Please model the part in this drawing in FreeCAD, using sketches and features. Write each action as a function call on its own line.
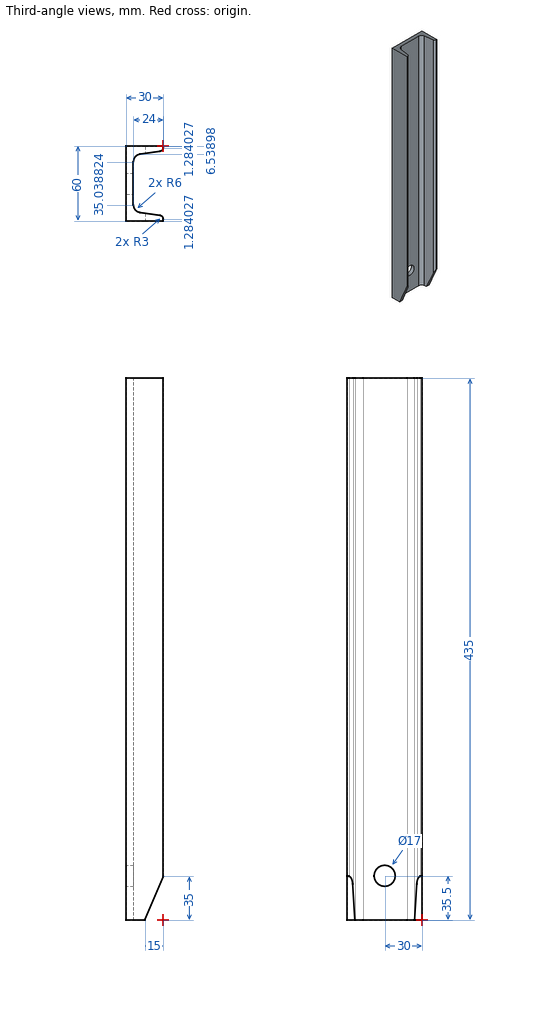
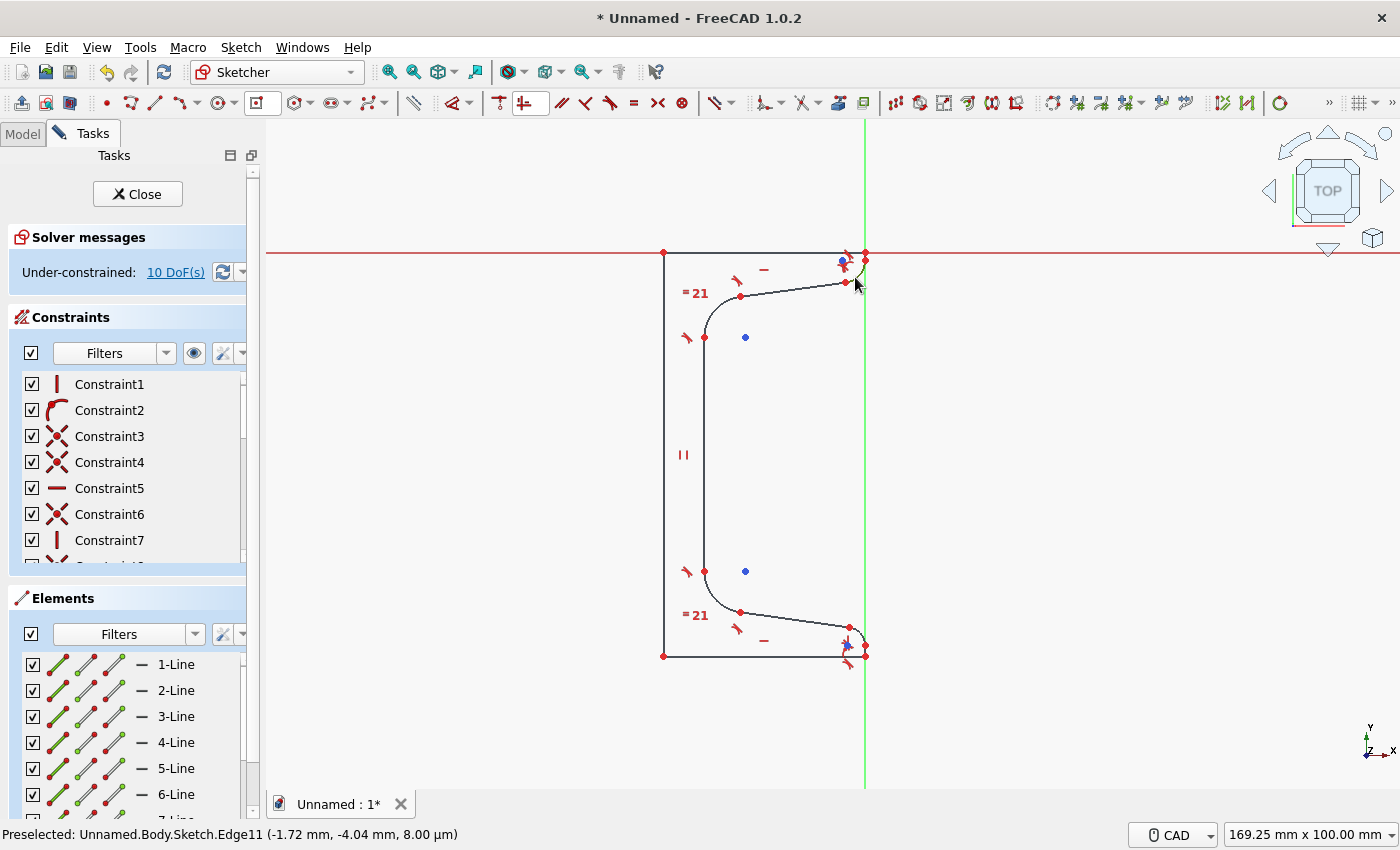
scroll(863, 638, up, 3)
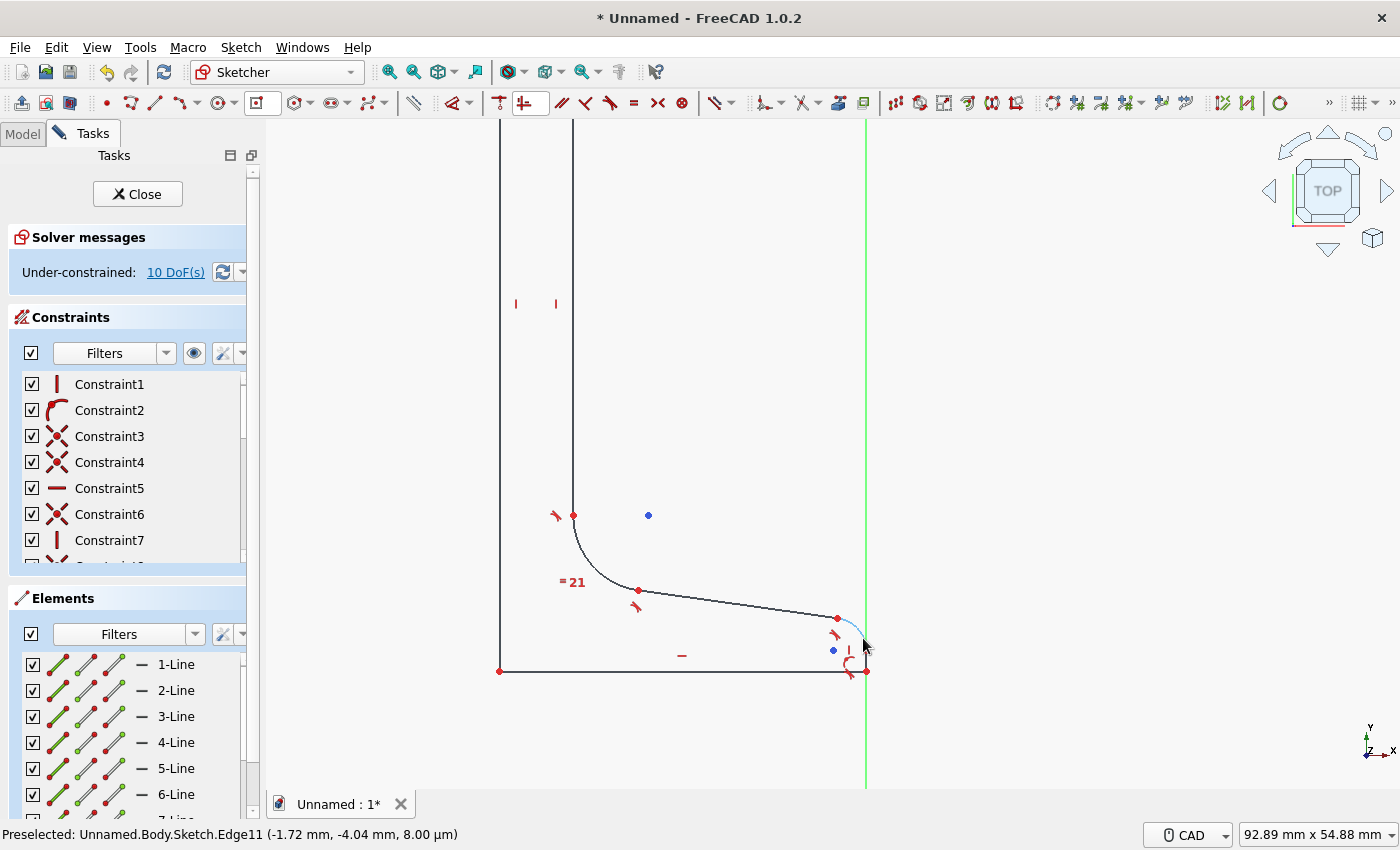
click(863, 637)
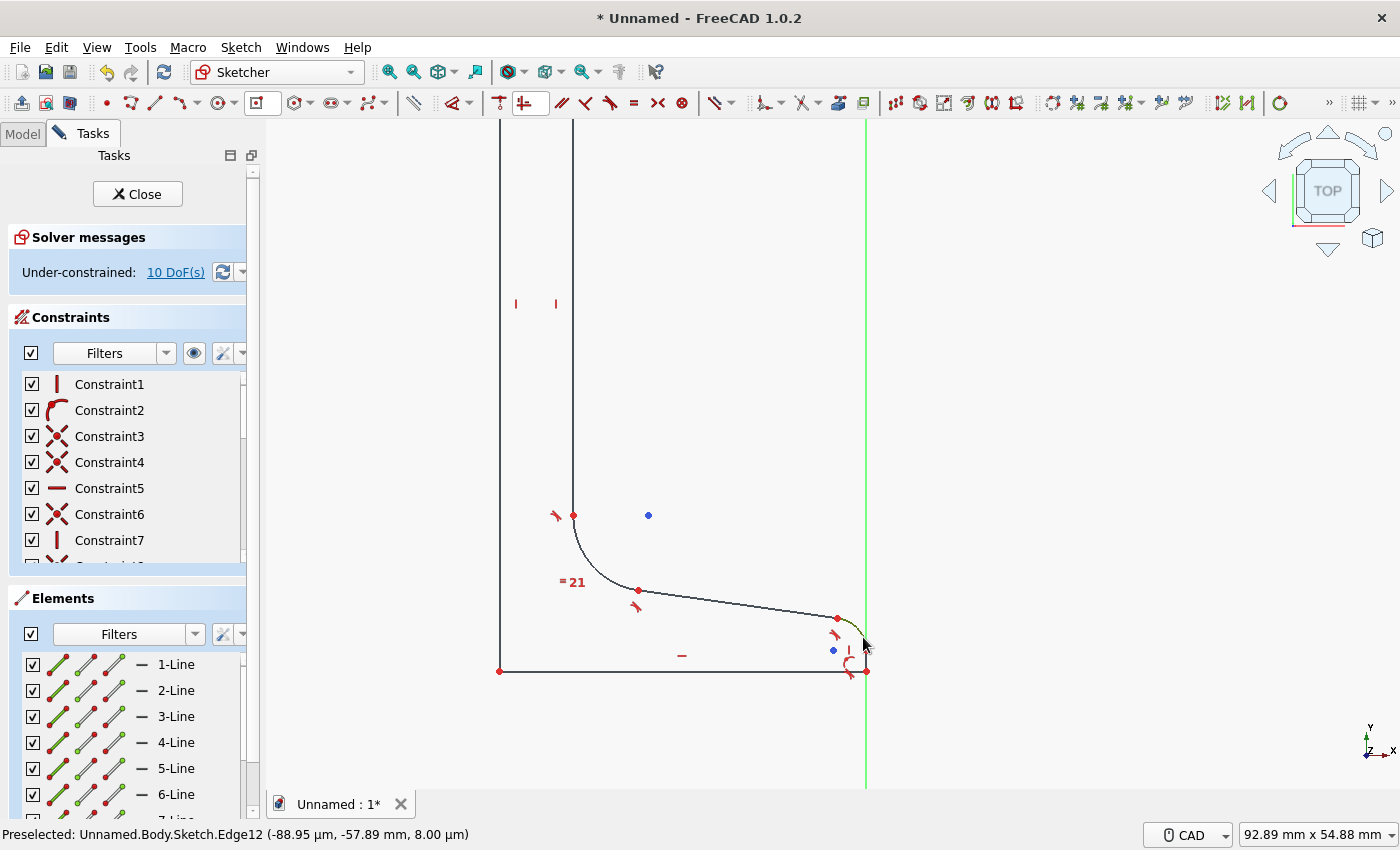
click(634, 104)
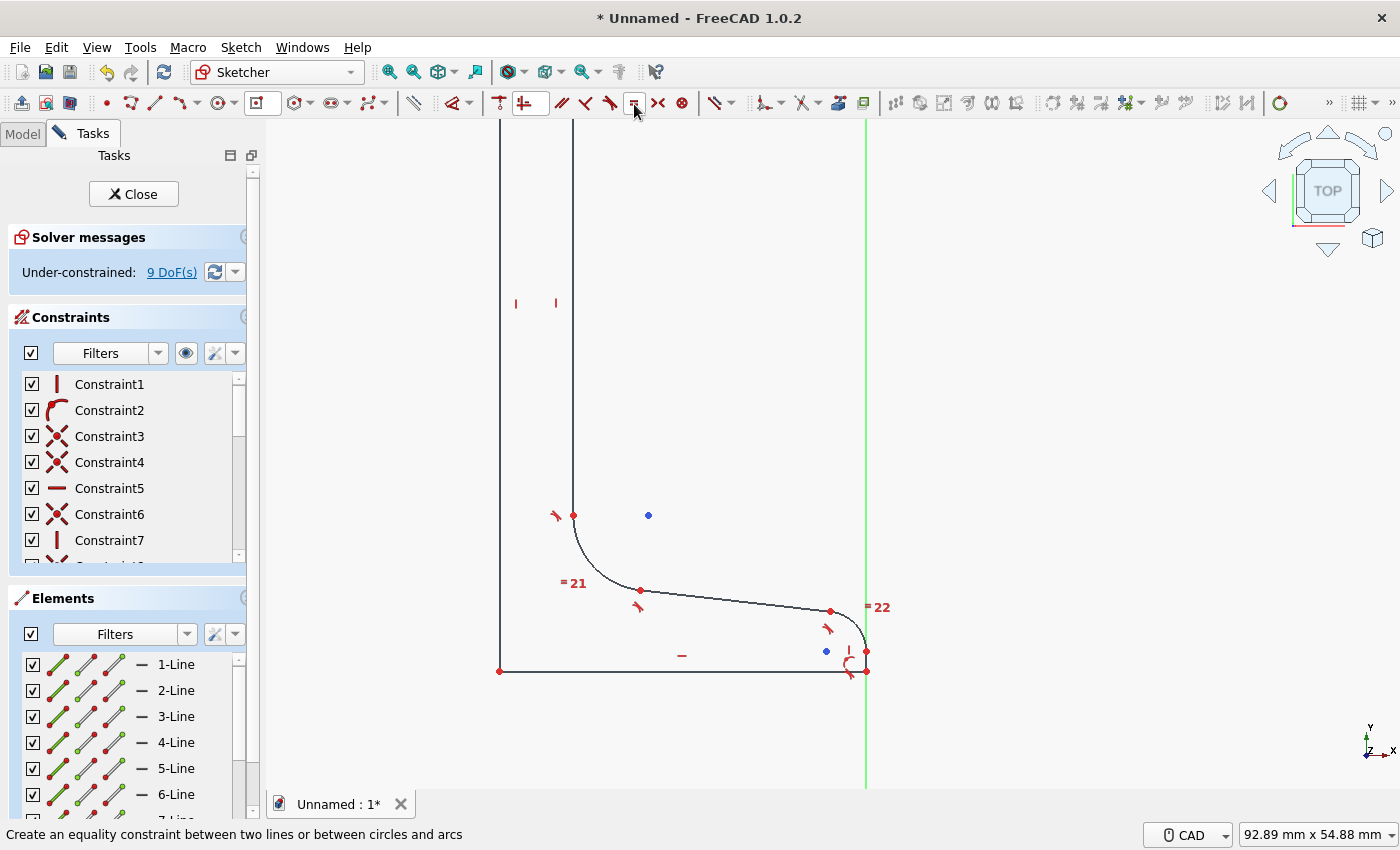
click(580, 547)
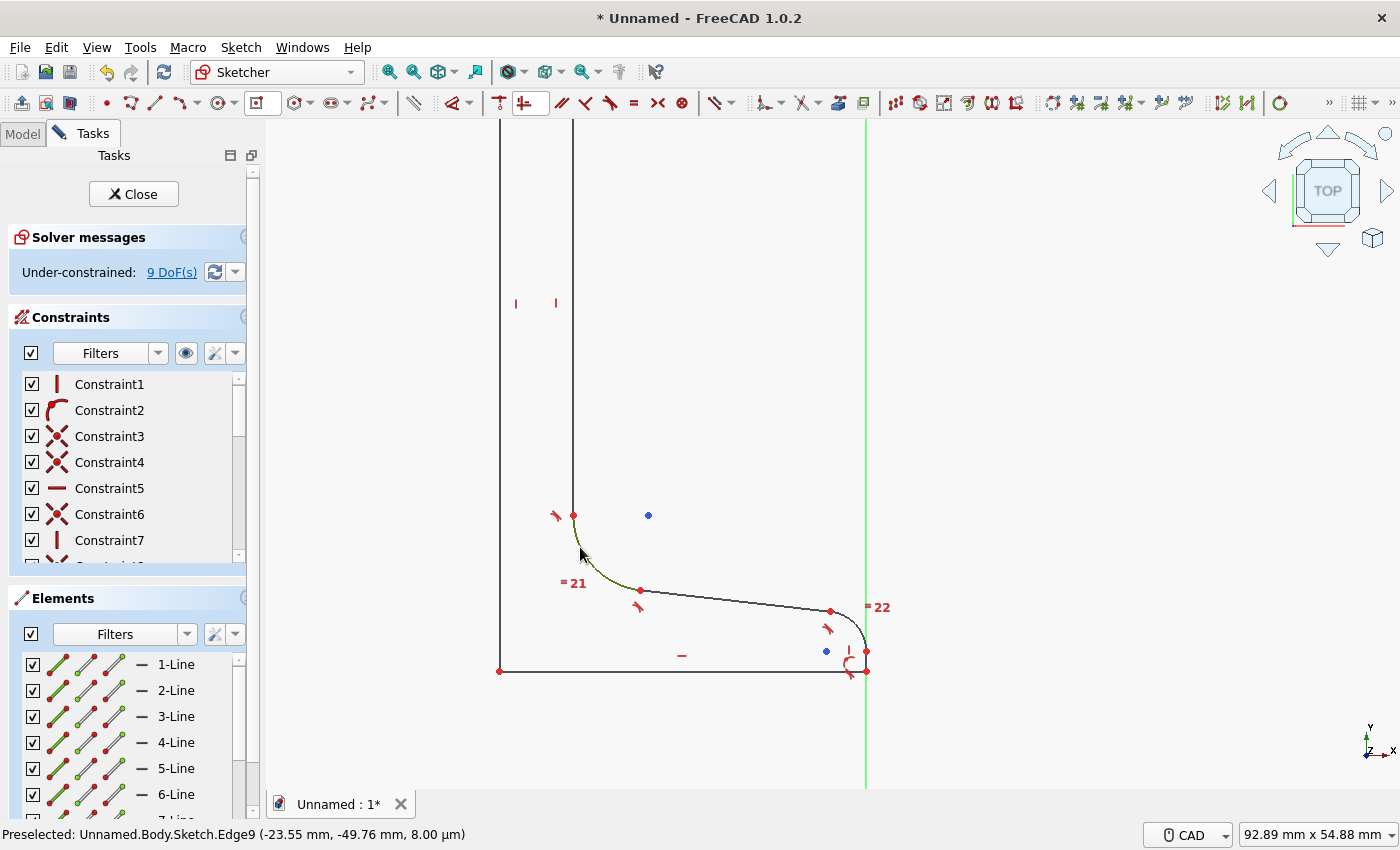
click(472, 104)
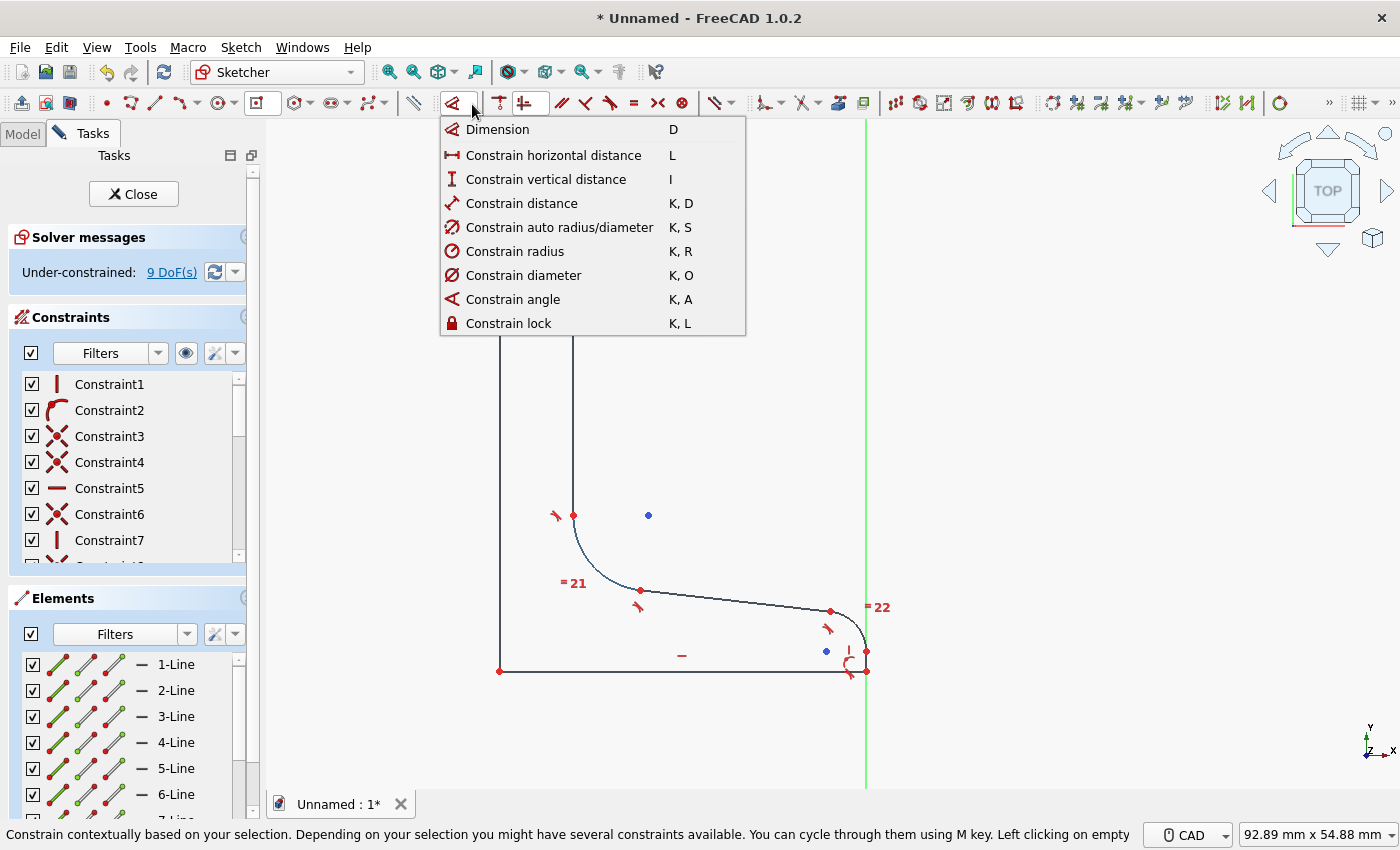
click(593, 251)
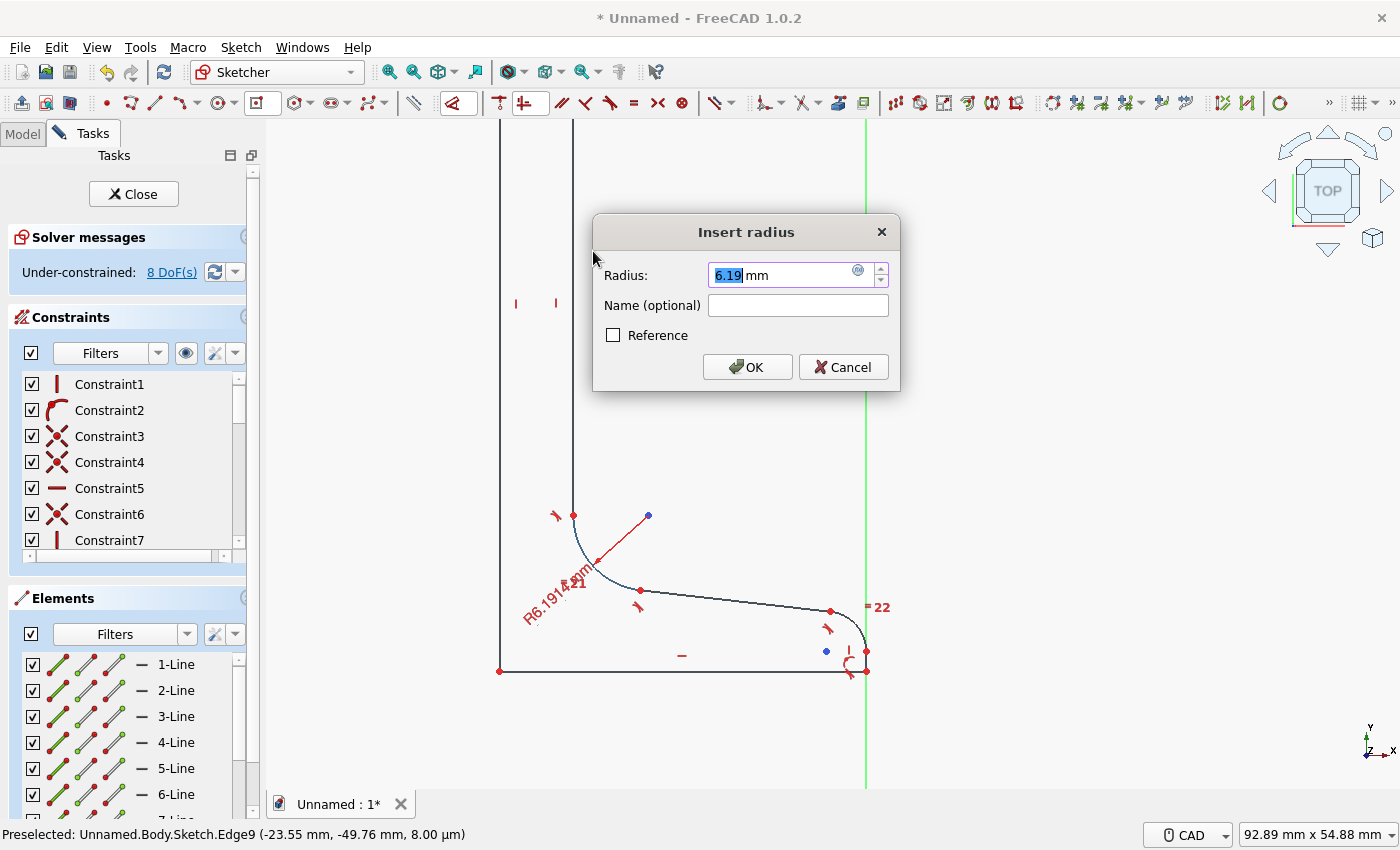
text(6)
key(Return)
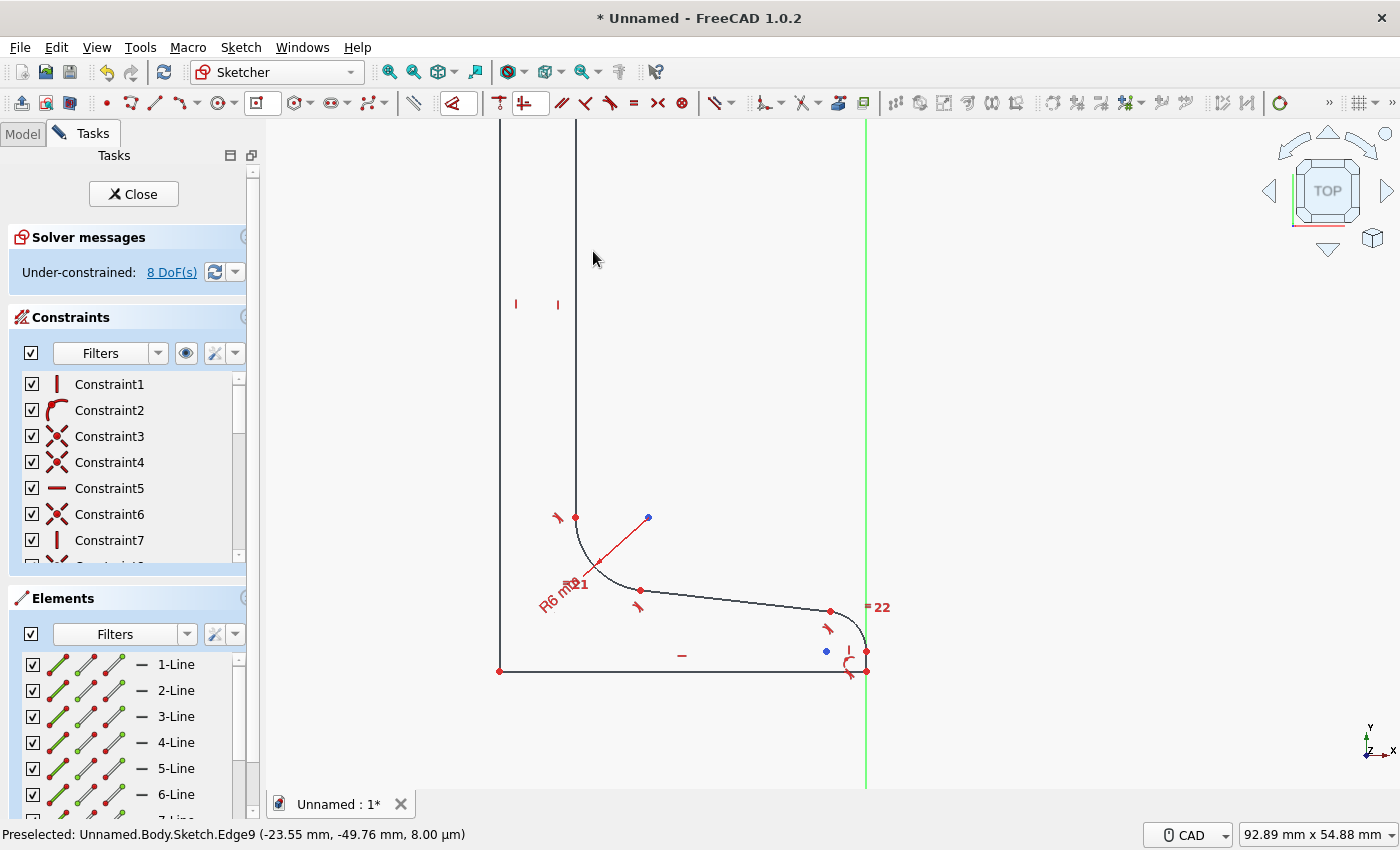
scroll(863, 639, down, 3)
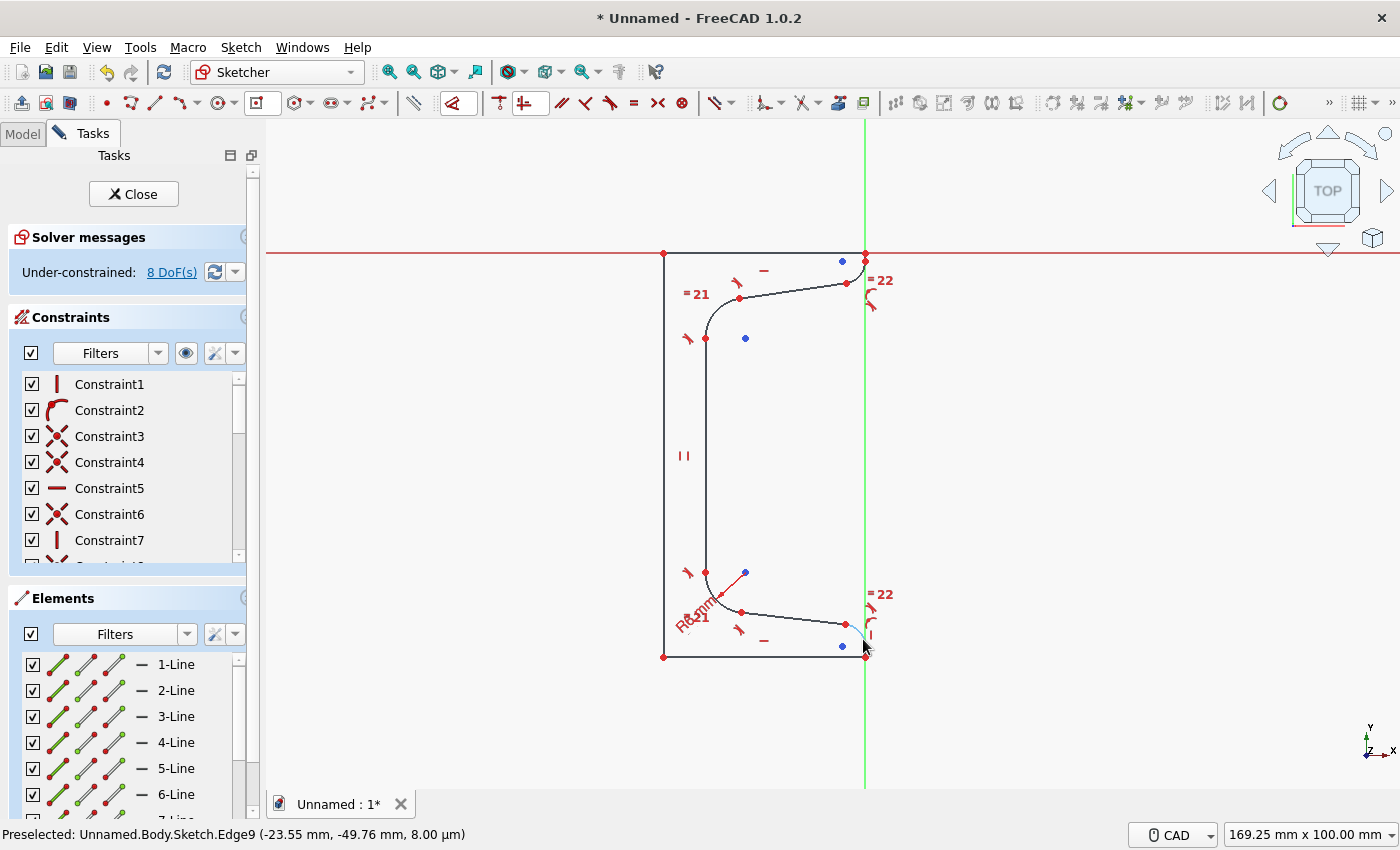
scroll(855, 280, up, 4)